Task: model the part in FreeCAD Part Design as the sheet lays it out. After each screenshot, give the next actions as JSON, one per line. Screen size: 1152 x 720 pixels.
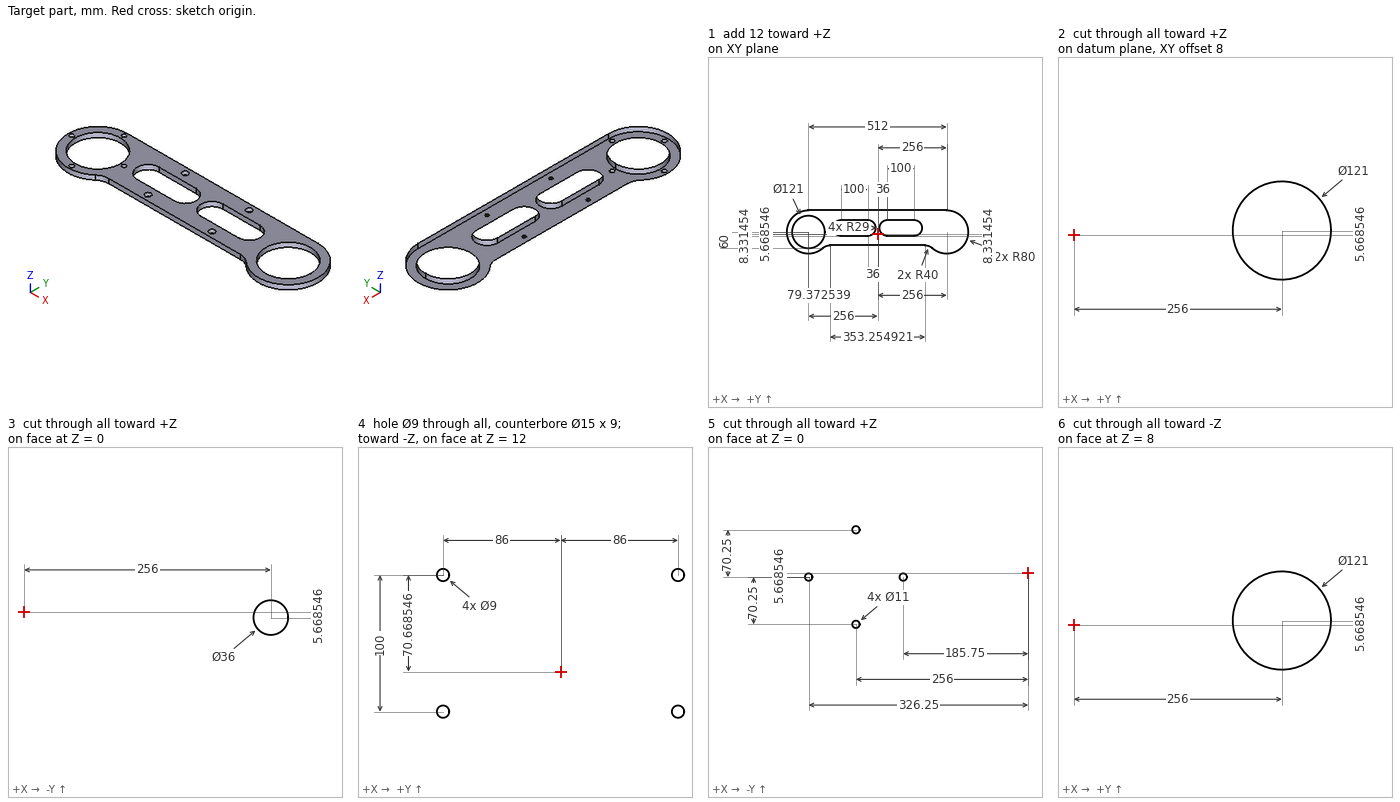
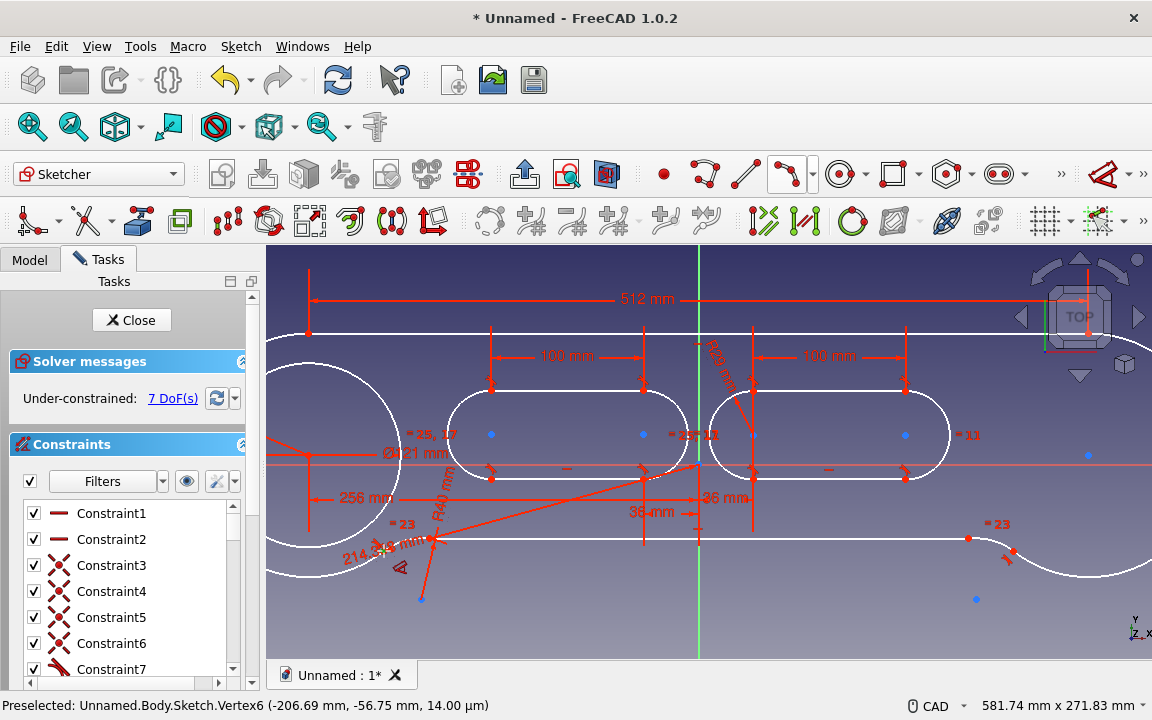
{"action": "left_click", "coordinate": [309, 455]}
{"action": "left_click", "coordinate": [418, 525]}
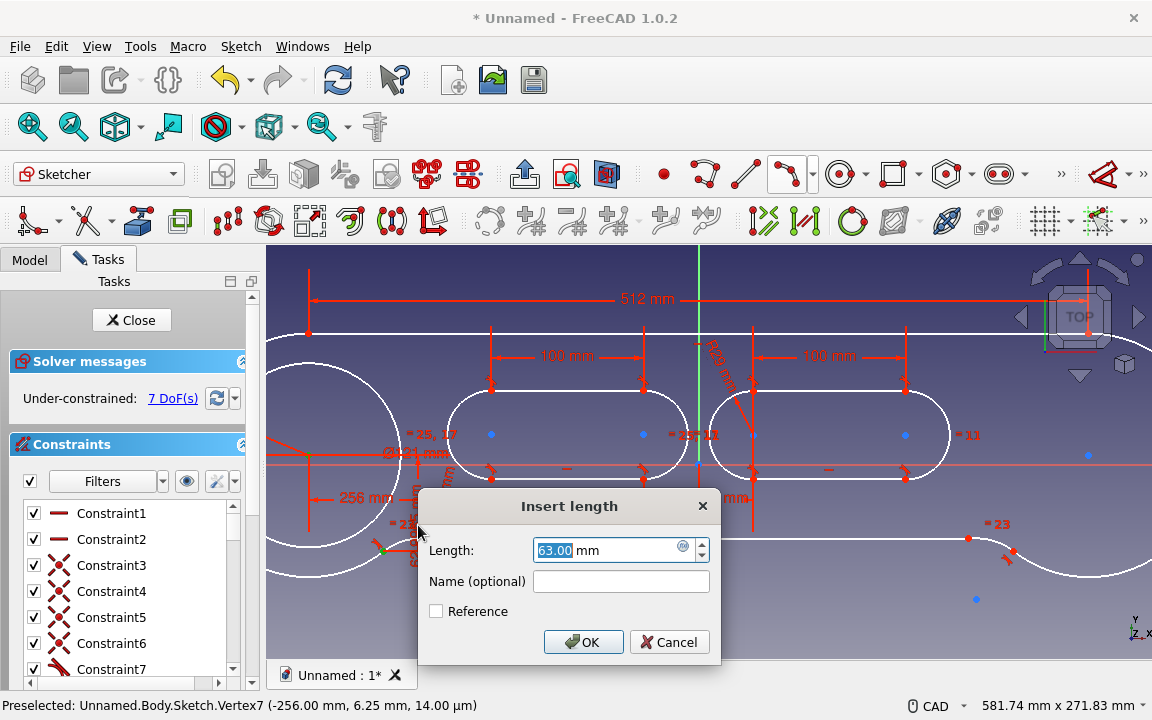
{"action": "type", "text": "60"}
{"action": "key", "text": "Return"}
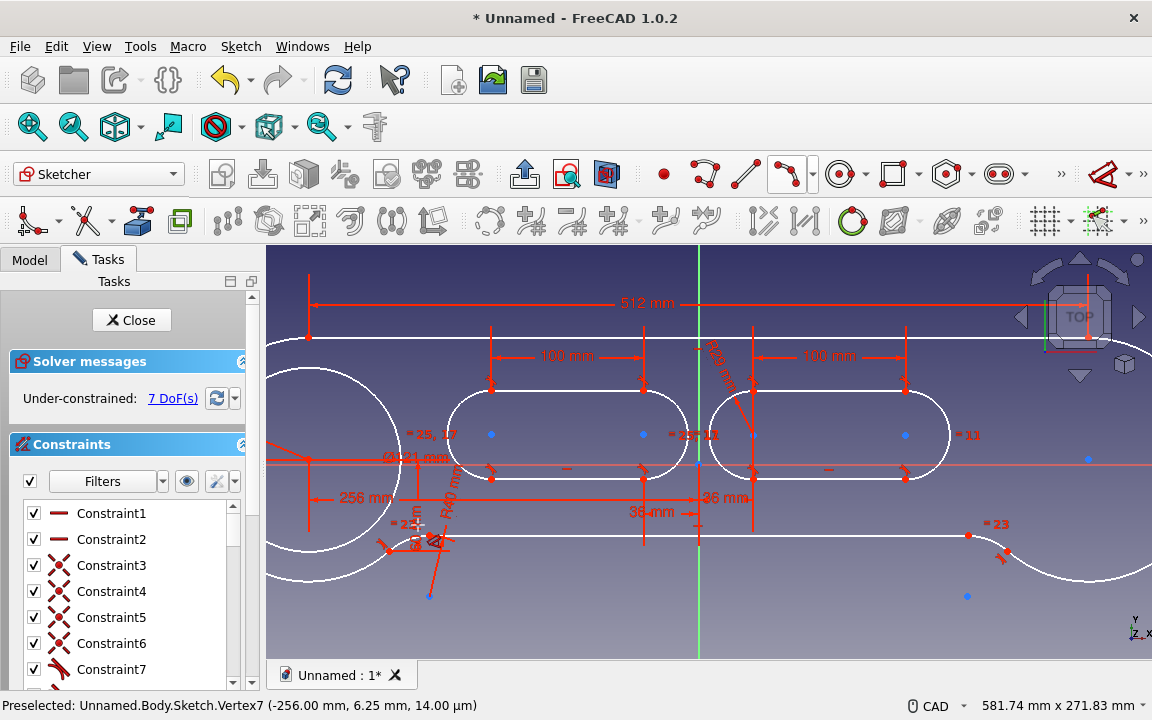
{"action": "scroll", "coordinate": [593, 461], "scroll_direction": "down", "scroll_amount": 4}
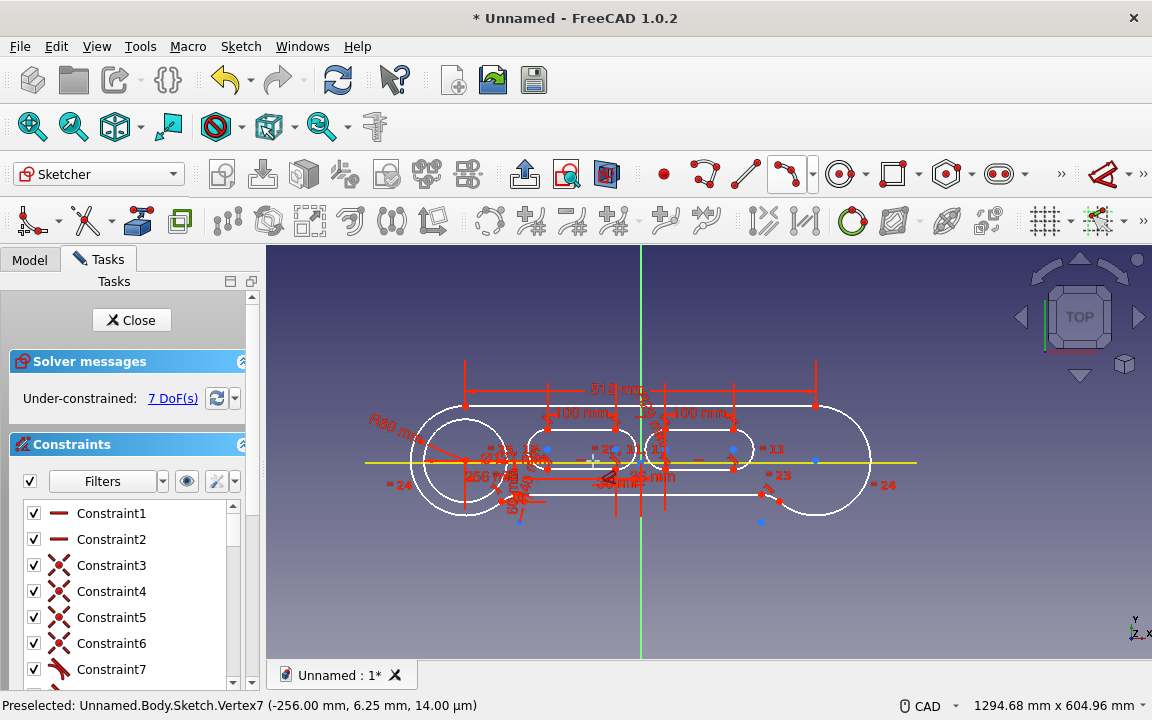
{"action": "left_click", "coordinate": [816, 406]}
{"action": "left_click", "coordinate": [728, 372]}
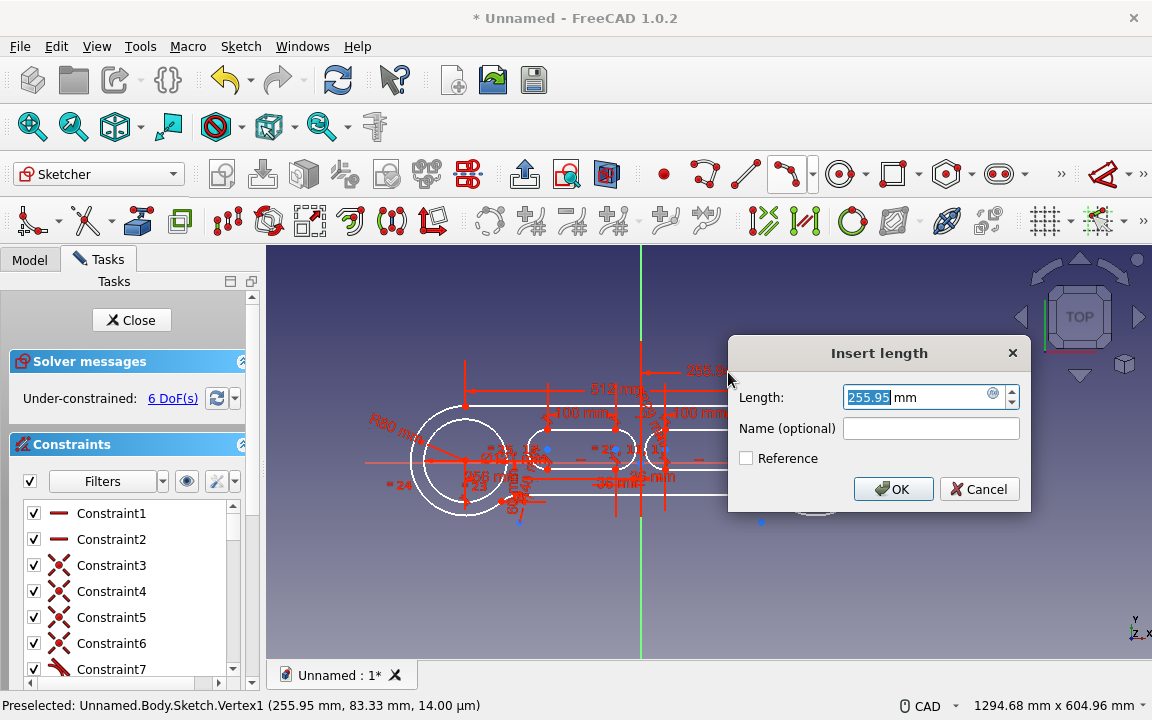
{"action": "type", "text": "256"}
{"action": "key", "text": "Return"}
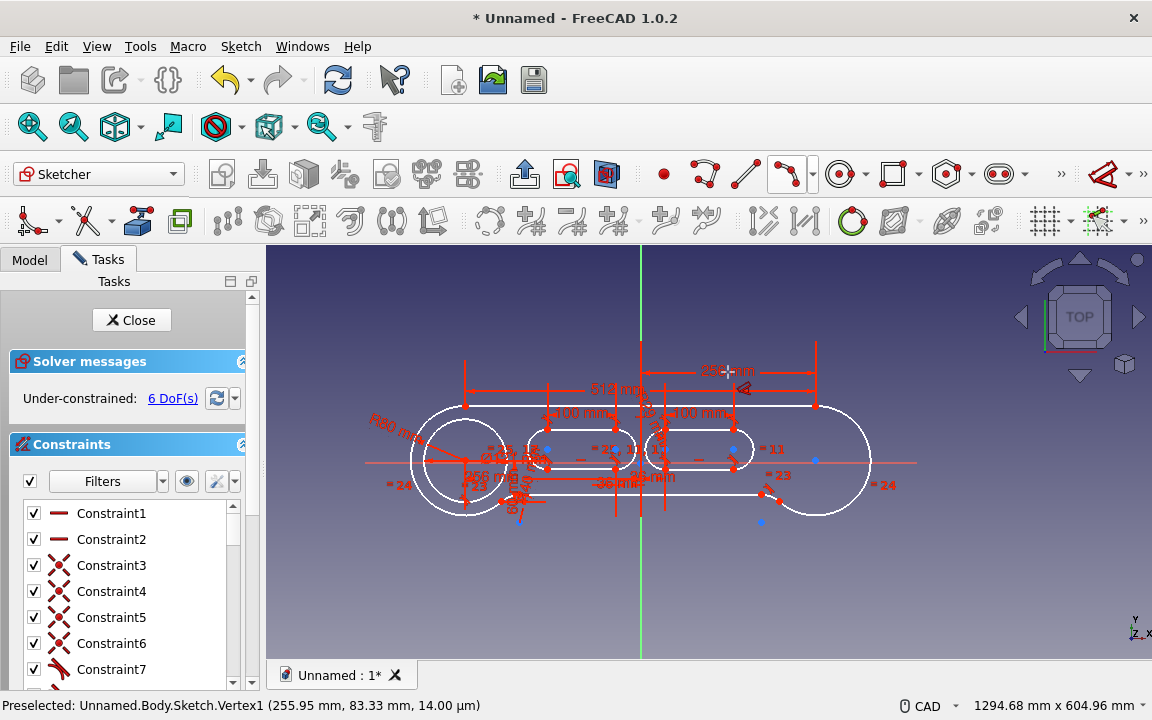
{"action": "left_click", "coordinate": [816, 461]}
{"action": "left_click", "coordinate": [790, 427]}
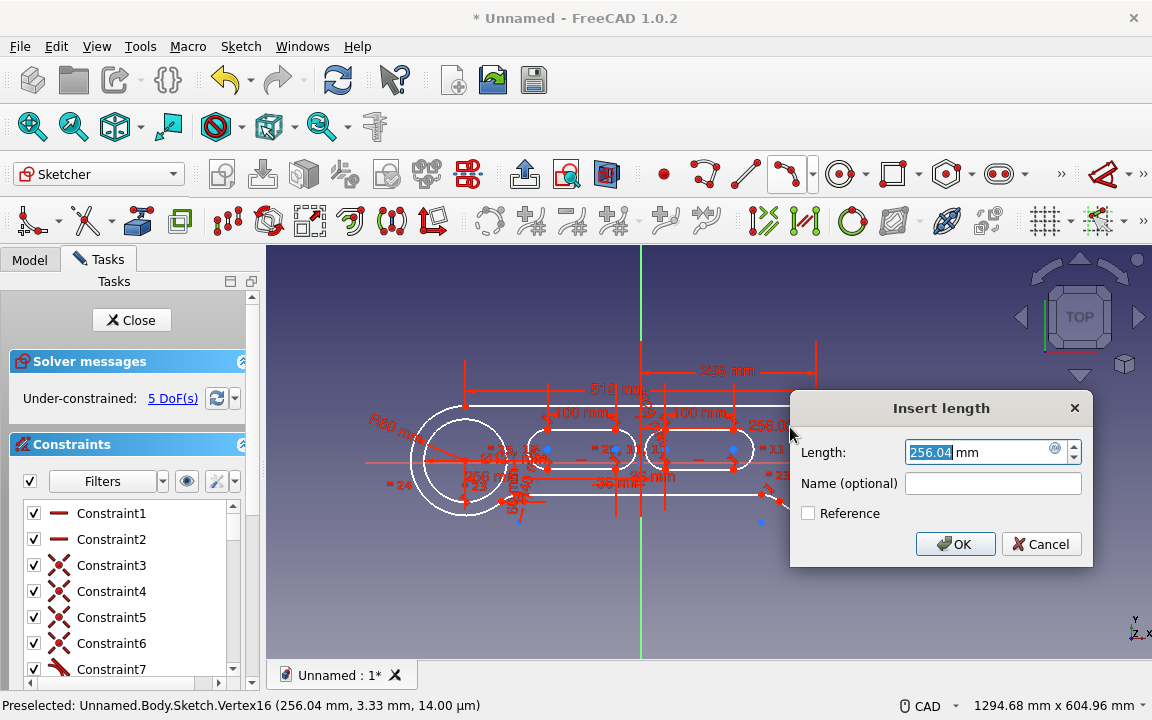
{"action": "type", "text": "256"}
{"action": "key", "text": "Return"}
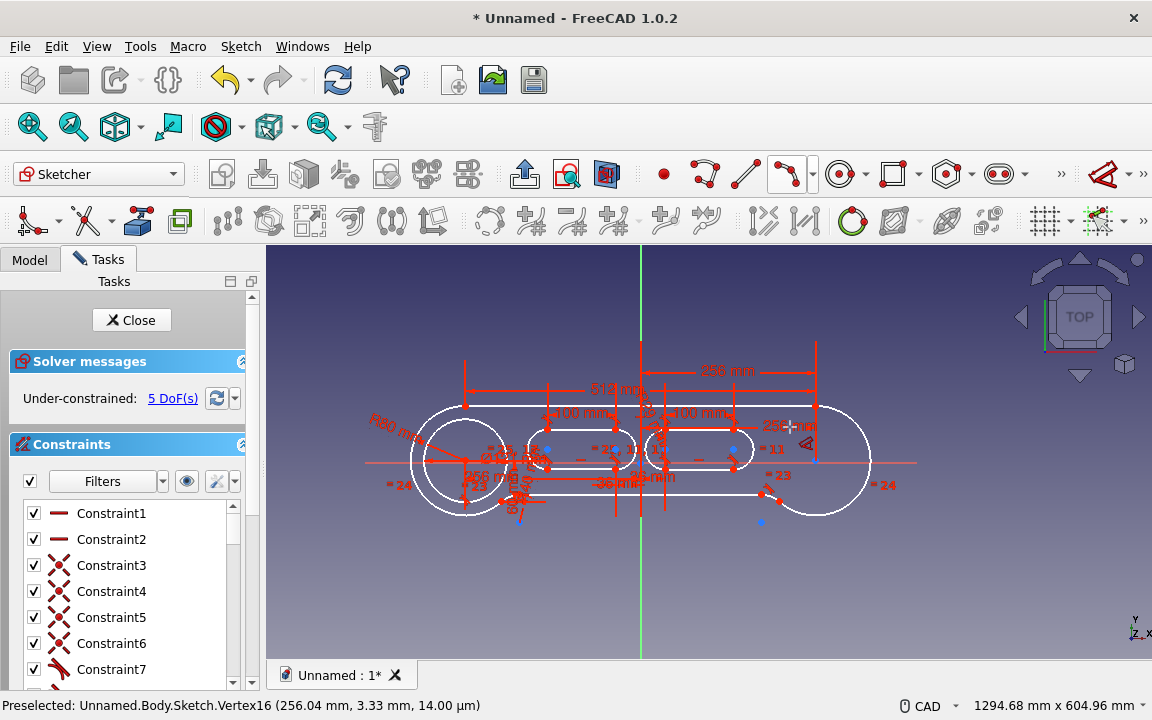
{"action": "scroll", "coordinate": [465, 461], "scroll_direction": "up", "scroll_amount": 12}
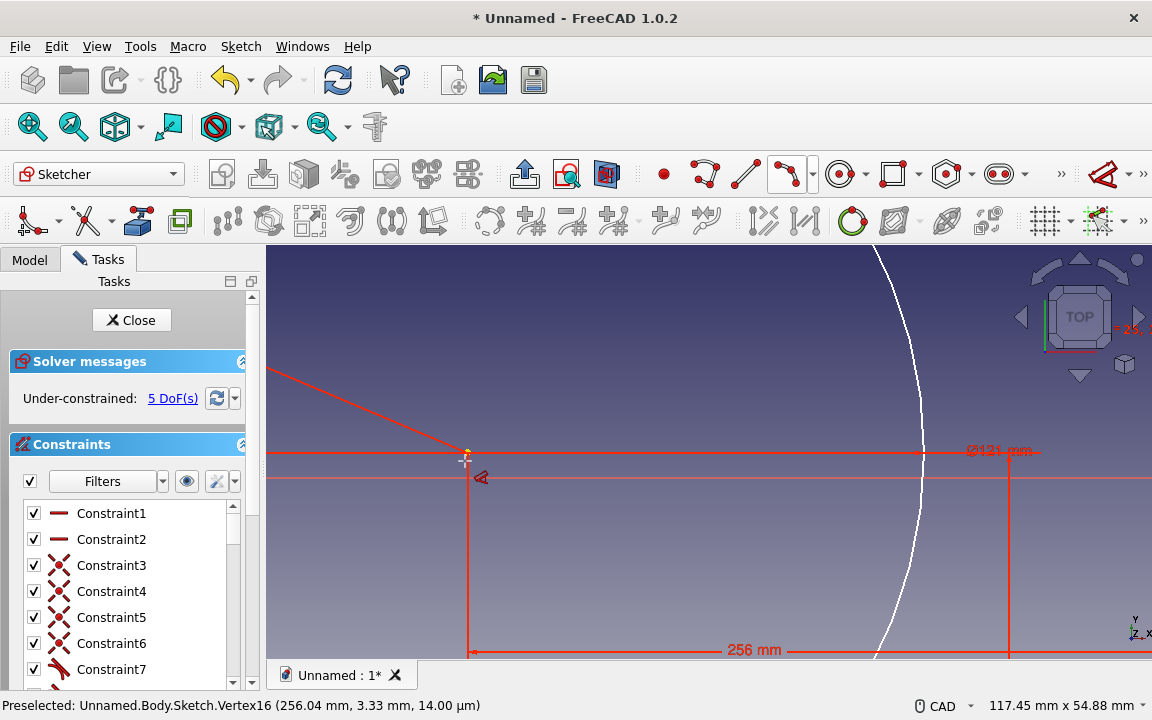
{"action": "left_click", "coordinate": [468, 453]}
{"action": "left_click", "coordinate": [434, 460]}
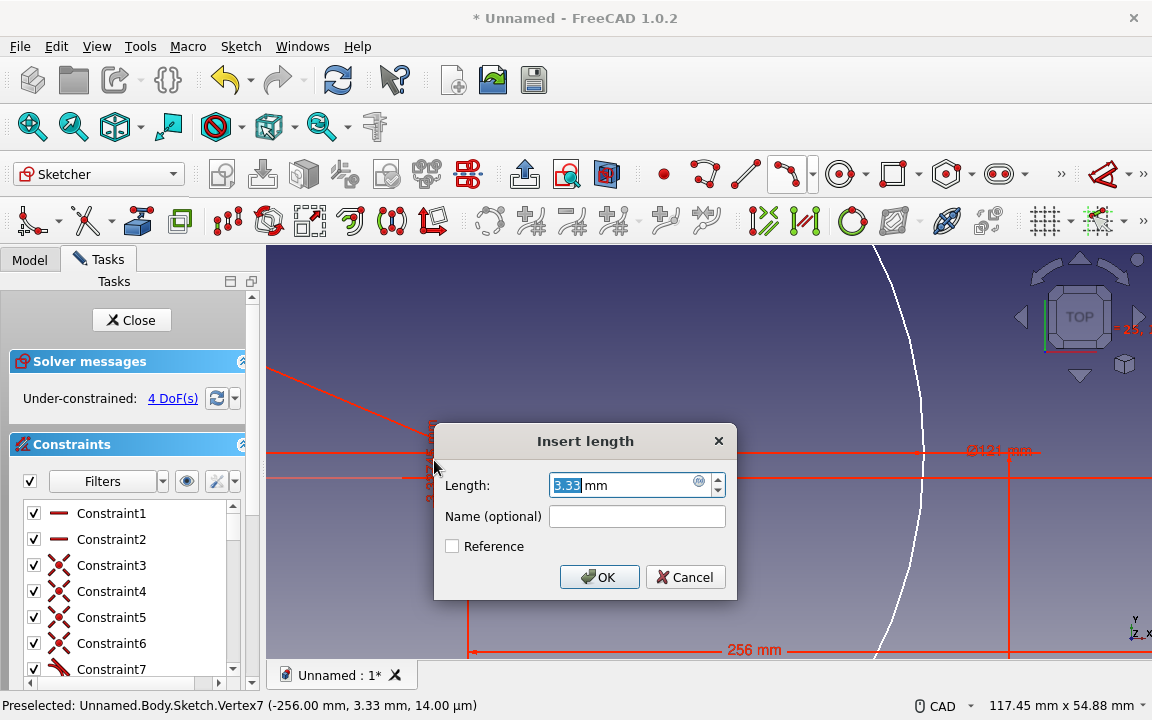
{"action": "type", "text": "5.668546"}
{"action": "key", "text": "Return"}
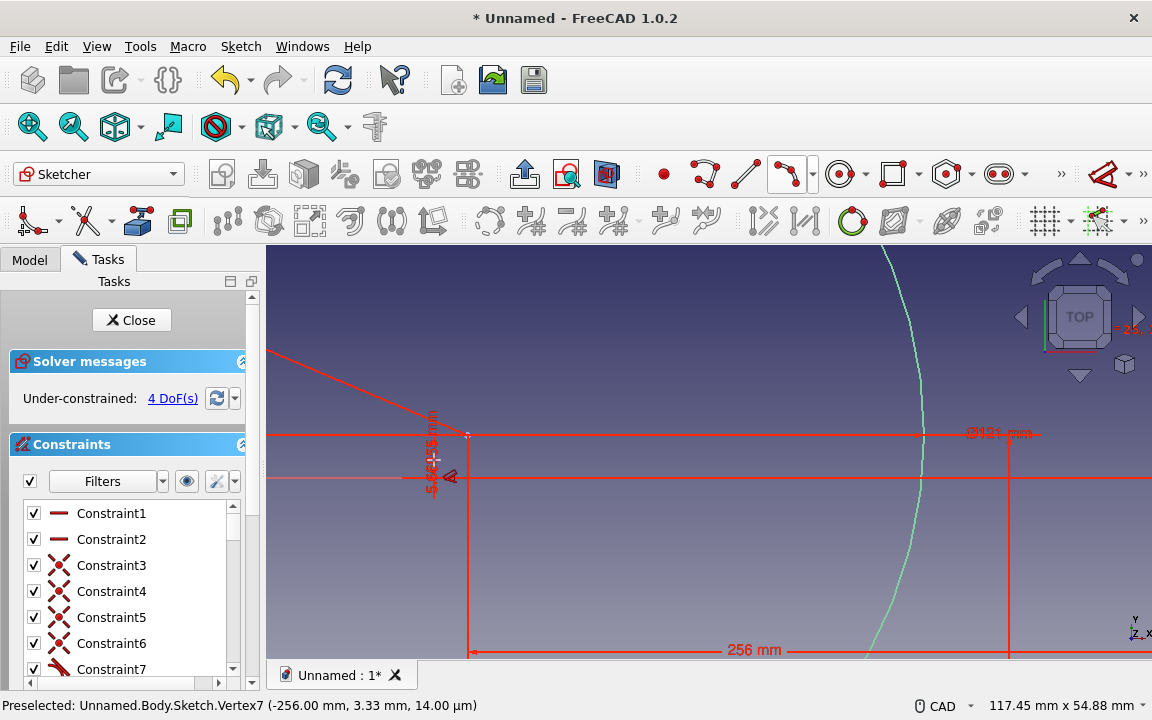
{"action": "scroll", "coordinate": [465, 461], "scroll_direction": "down", "scroll_amount": 12}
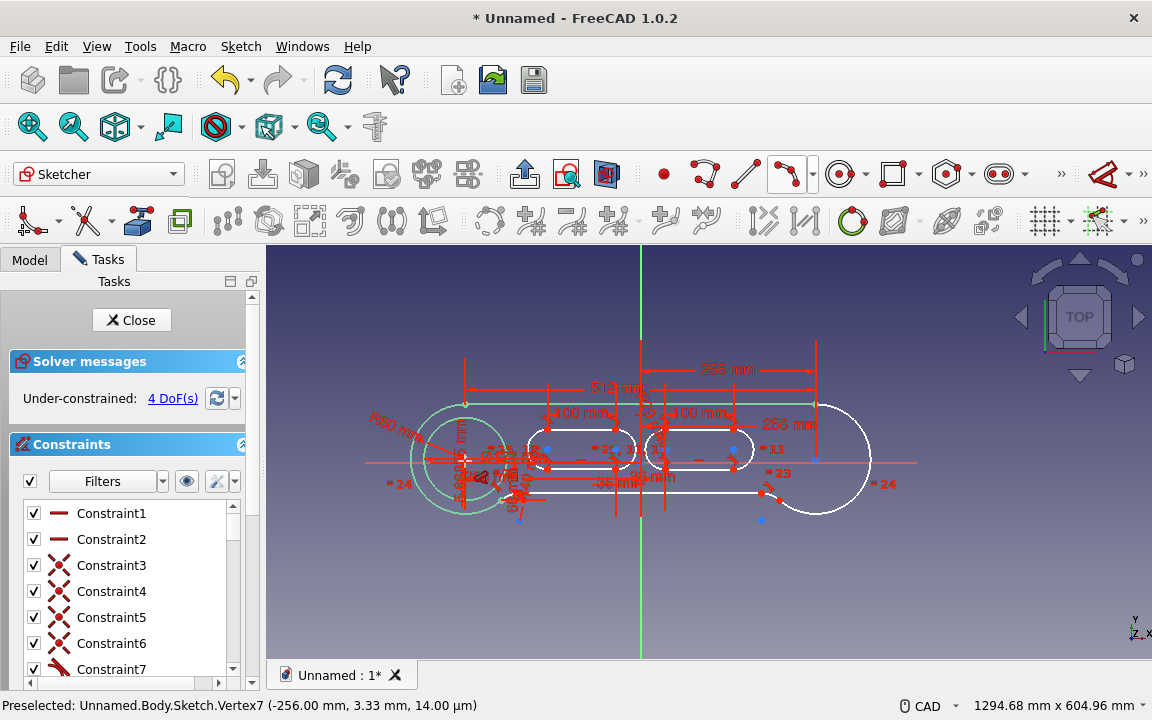
{"action": "scroll", "coordinate": [665, 470], "scroll_direction": "up", "scroll_amount": 10}